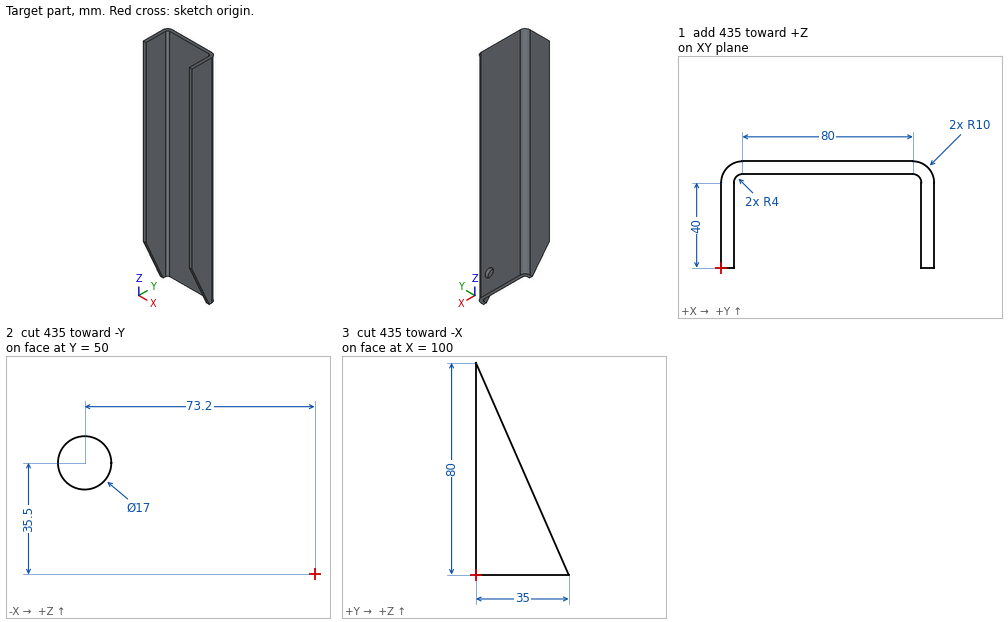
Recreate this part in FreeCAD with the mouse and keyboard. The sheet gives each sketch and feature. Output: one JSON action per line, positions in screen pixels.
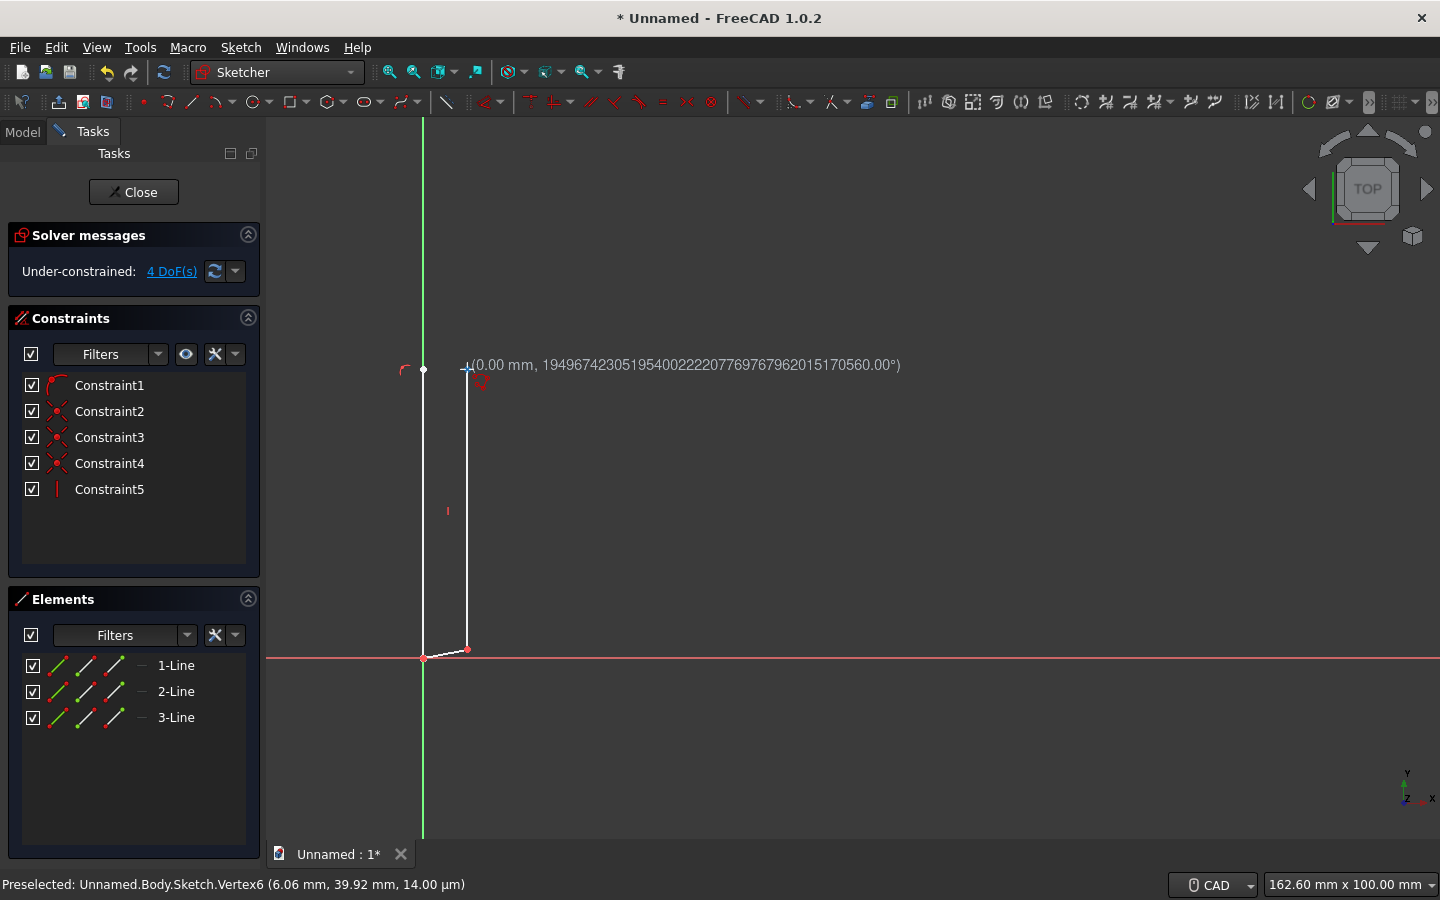
{"action": "left_click", "coordinate": [192, 102]}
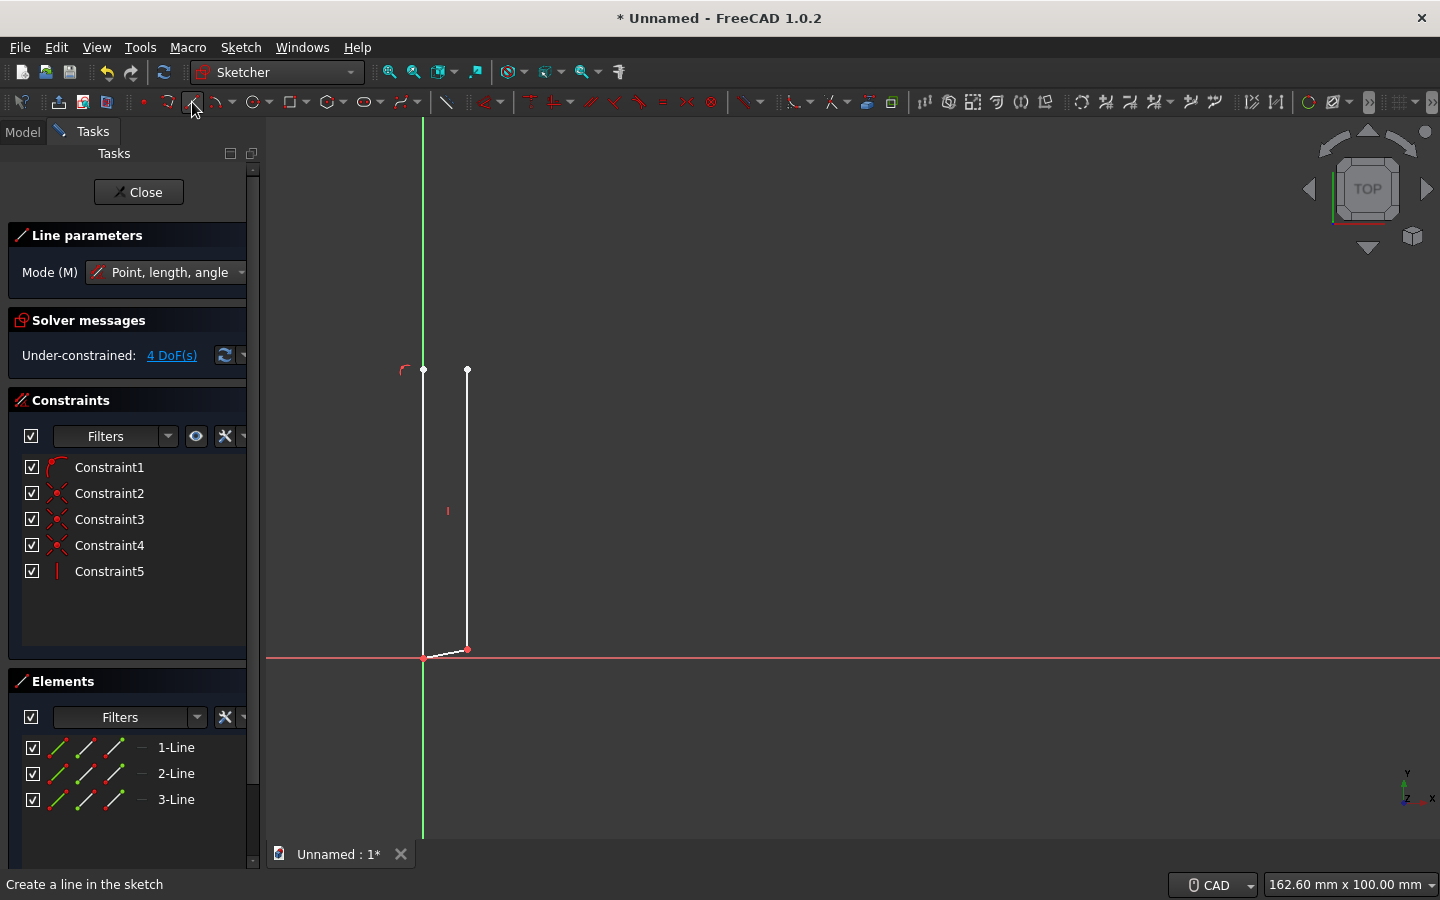
{"action": "left_click", "coordinate": [495, 341]}
{"action": "left_click", "coordinate": [1073, 341]}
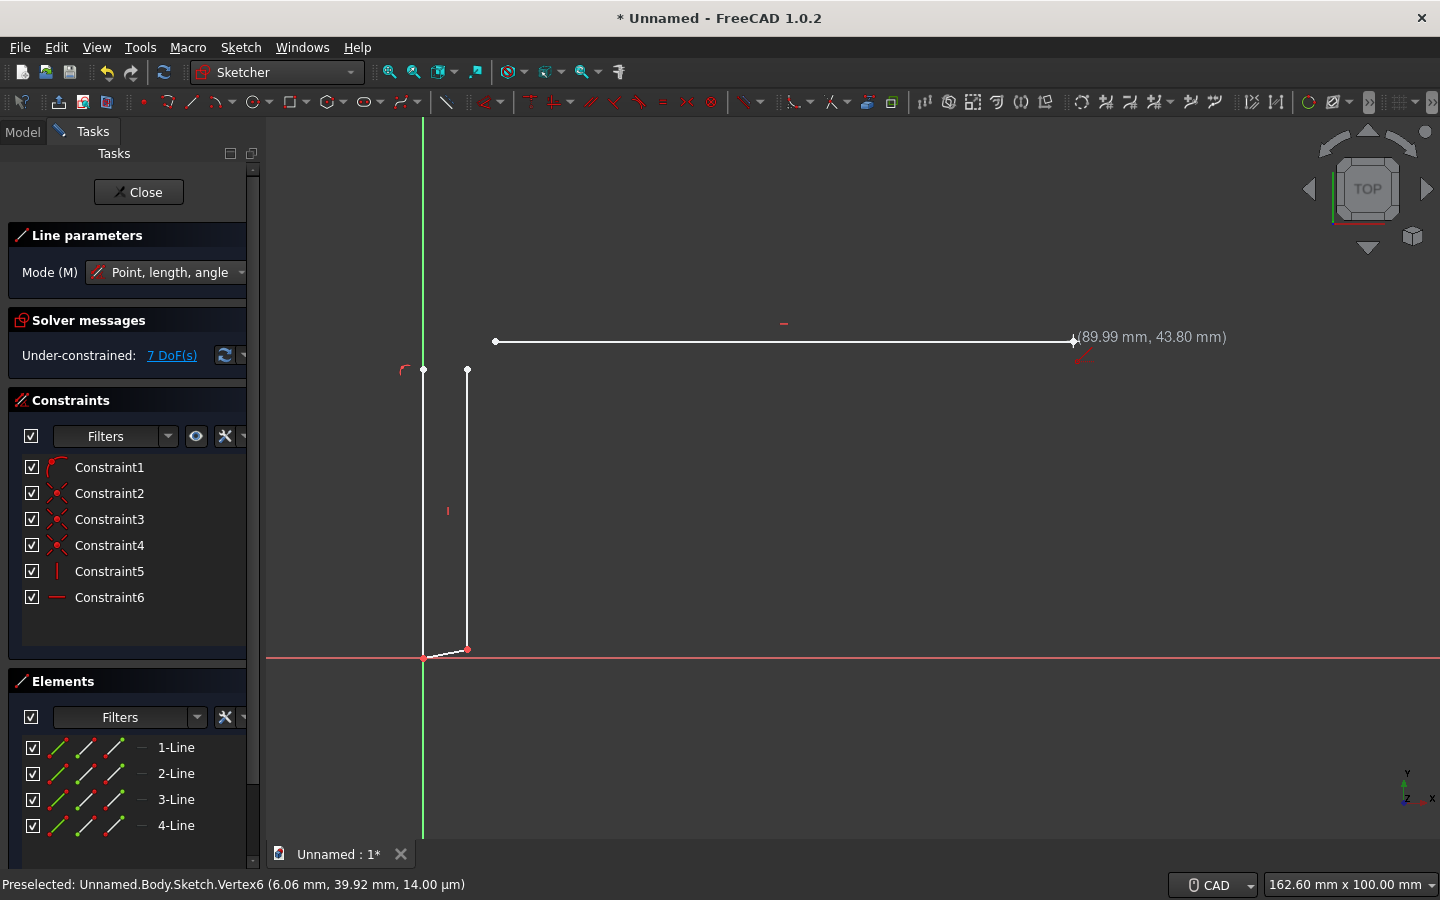
{"action": "left_click", "coordinate": [168, 102]}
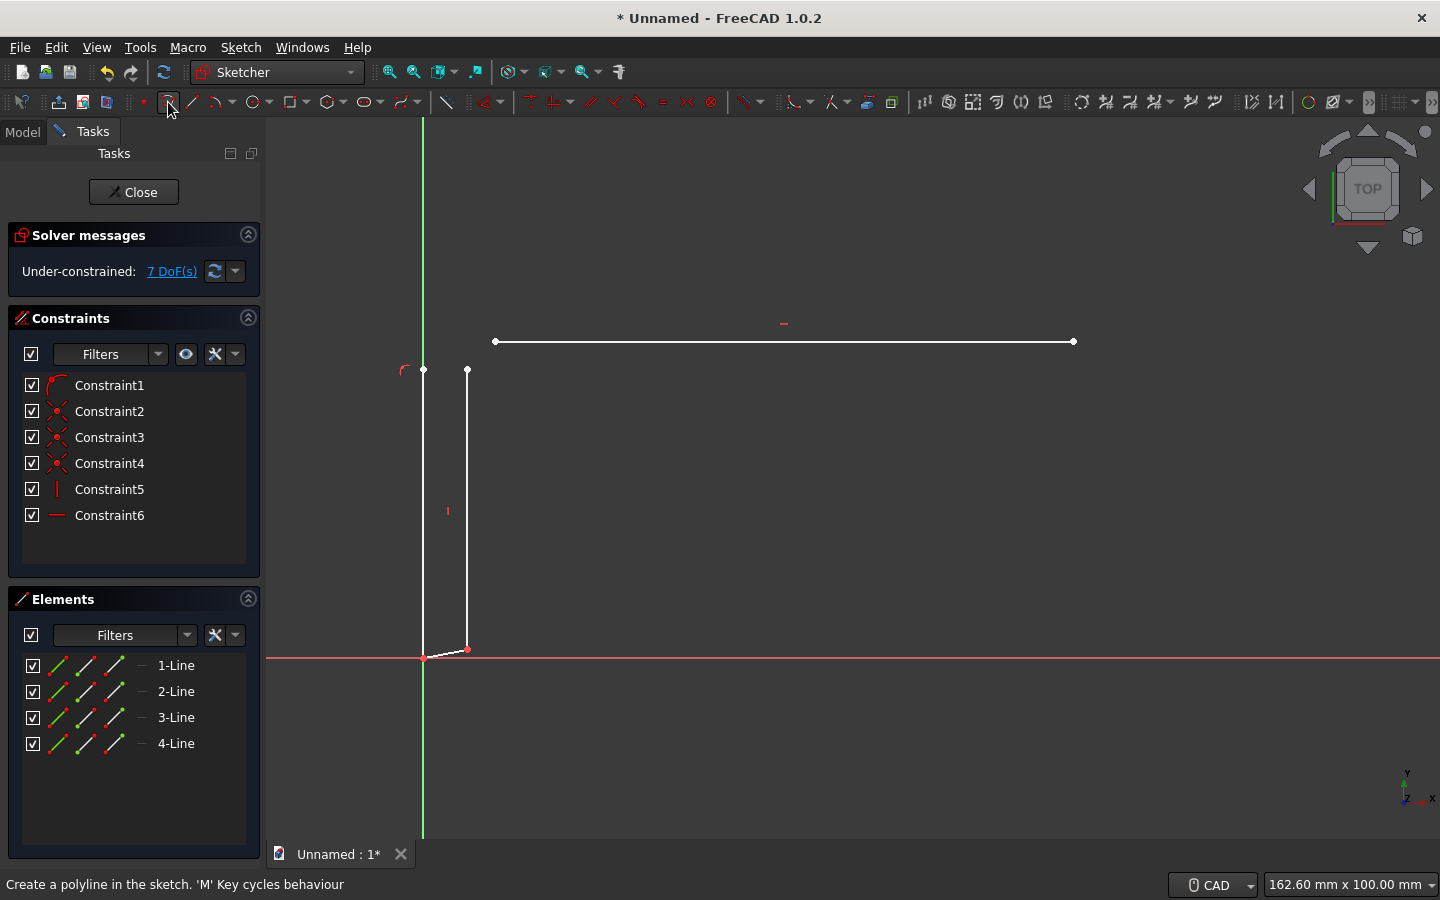
{"action": "left_click", "coordinate": [1102, 369]}
{"action": "left_click", "coordinate": [1102, 658]}
{"action": "left_click", "coordinate": [1145, 649]}
{"action": "left_click", "coordinate": [1145, 369]}
{"action": "right_click", "coordinate": [1145, 369]}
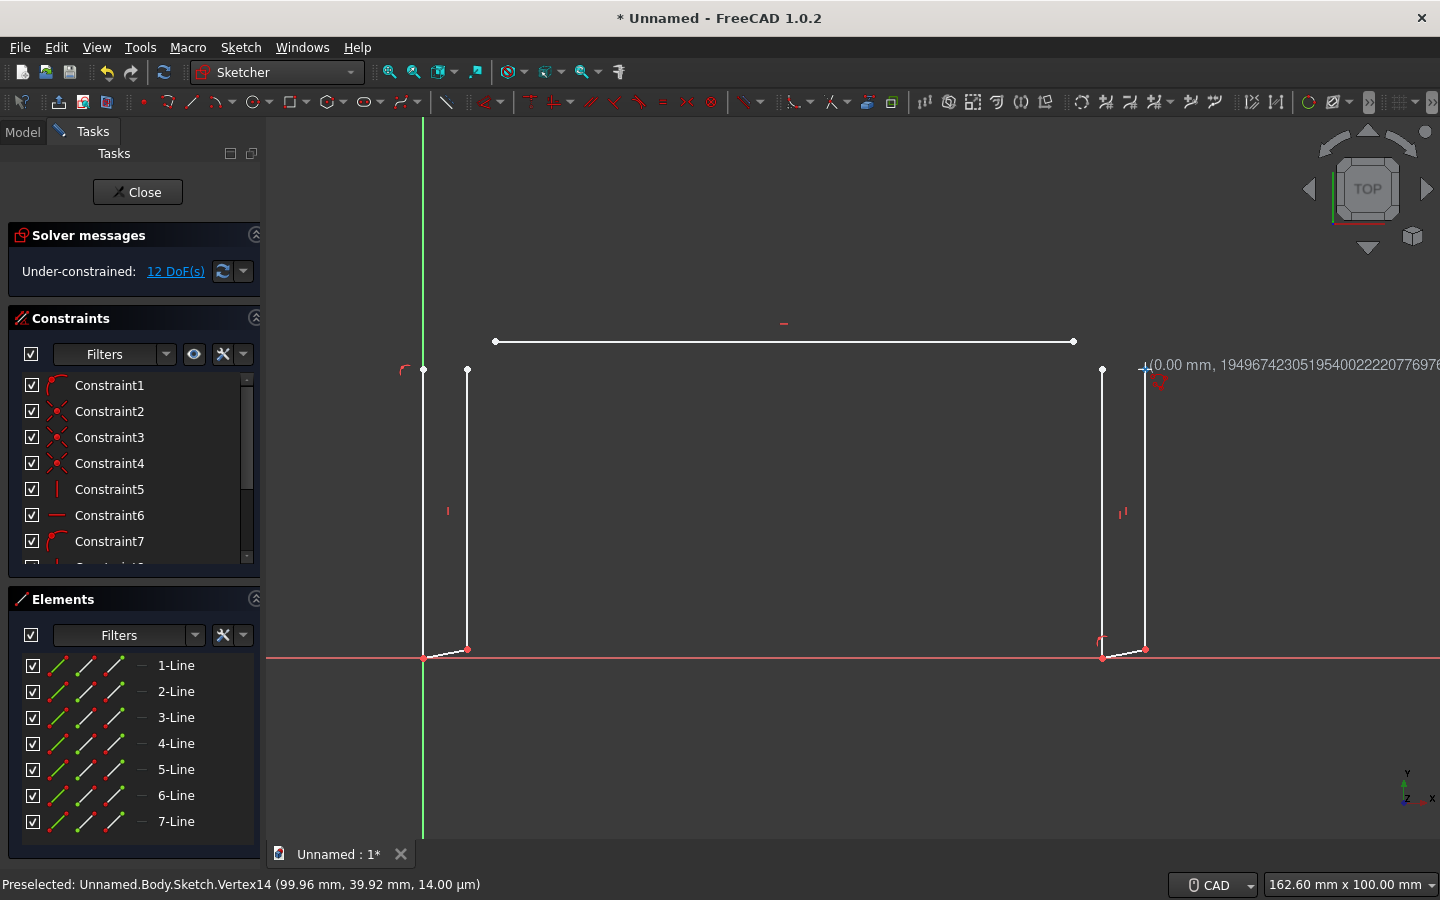
{"action": "left_click", "coordinate": [192, 102]}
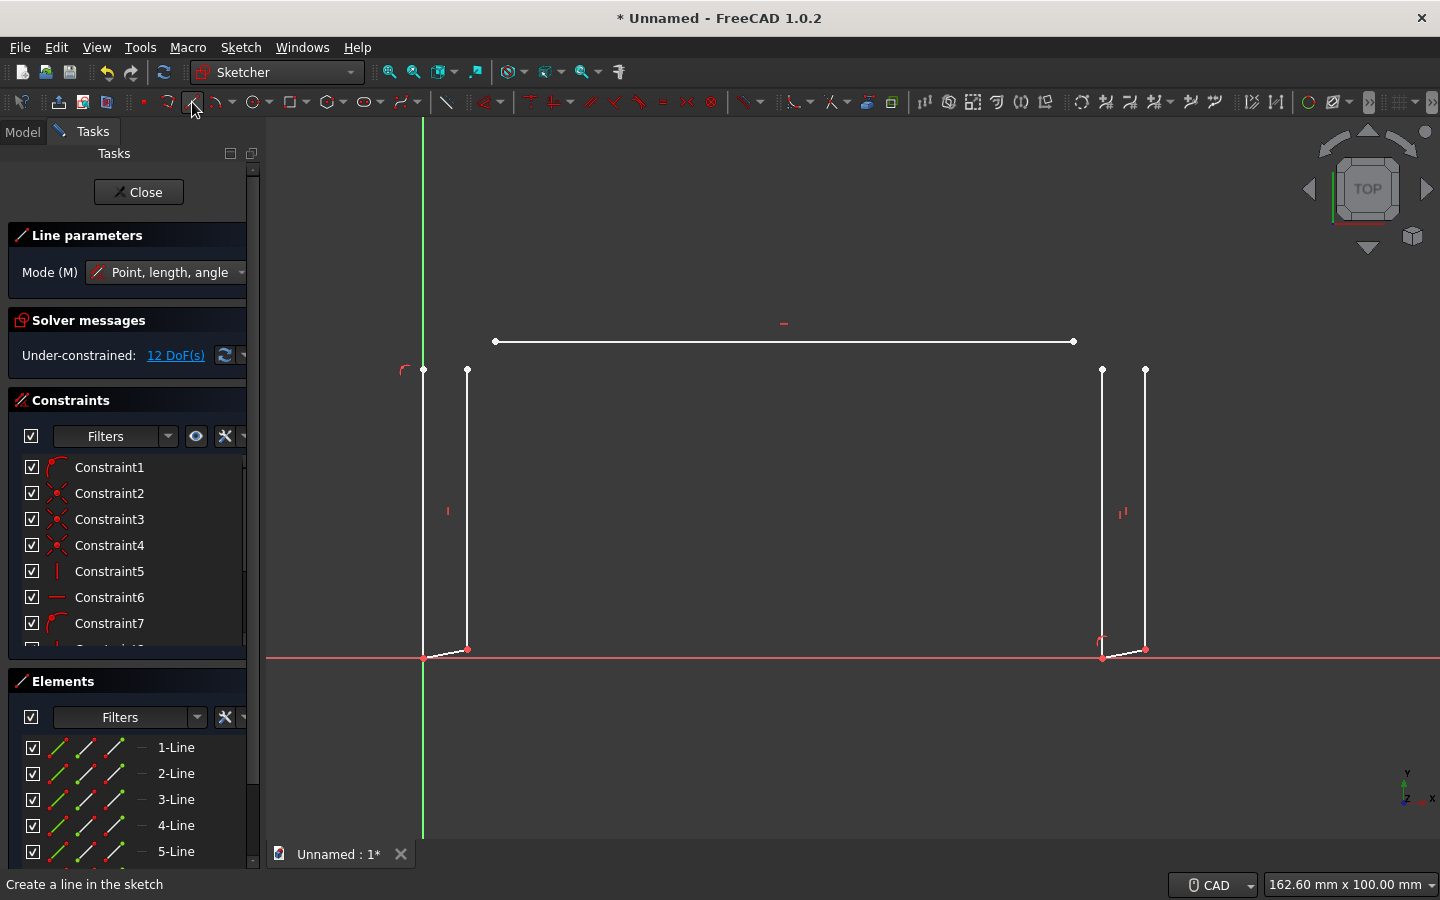
{"action": "left_click", "coordinate": [1073, 297]}
{"action": "left_click", "coordinate": [495, 297]}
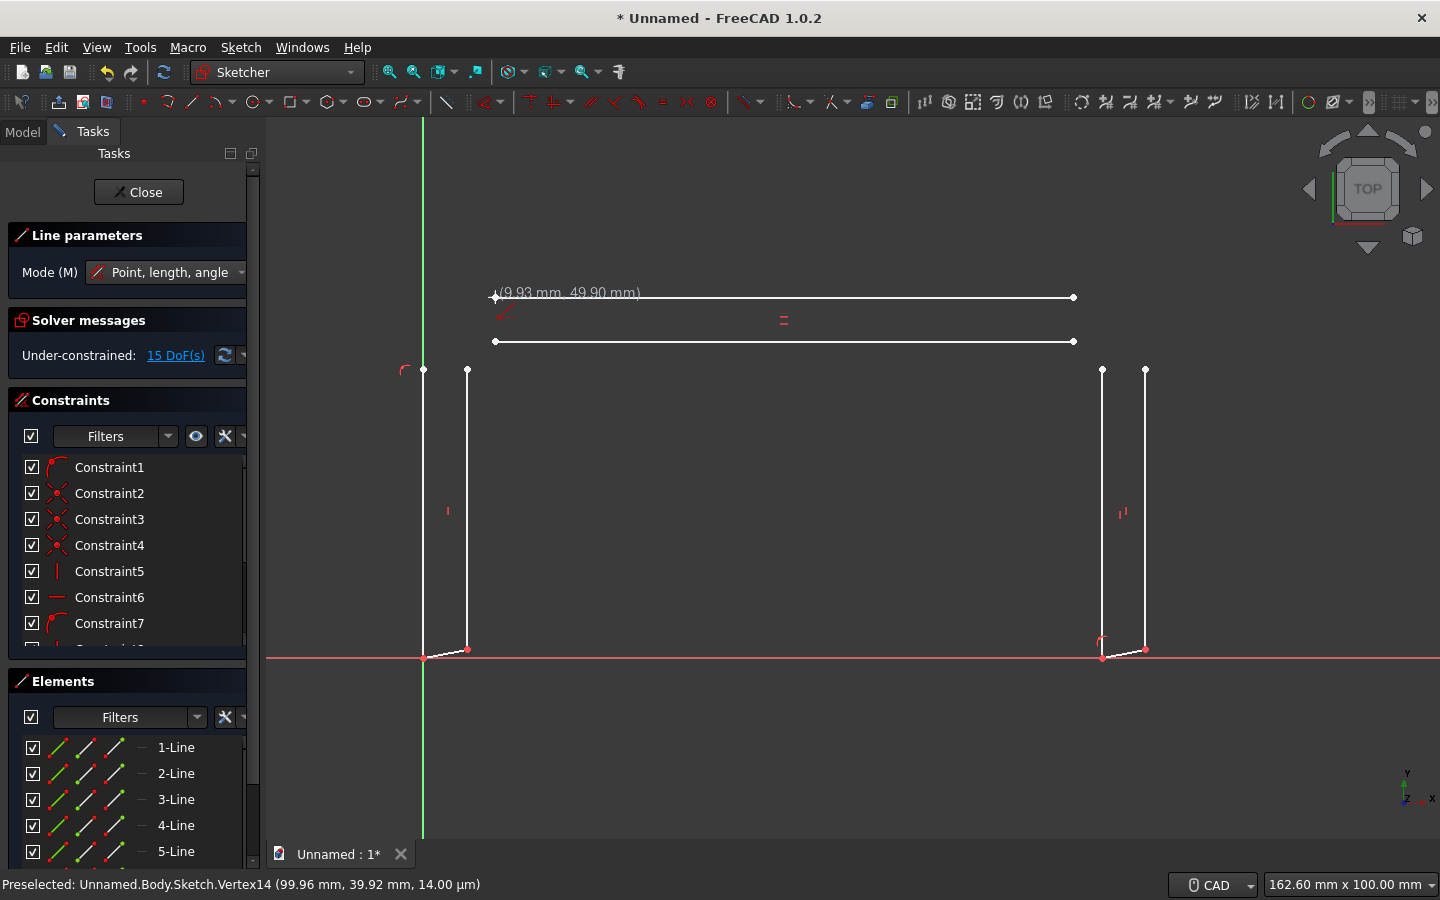
{"action": "left_click", "coordinate": [234, 102]}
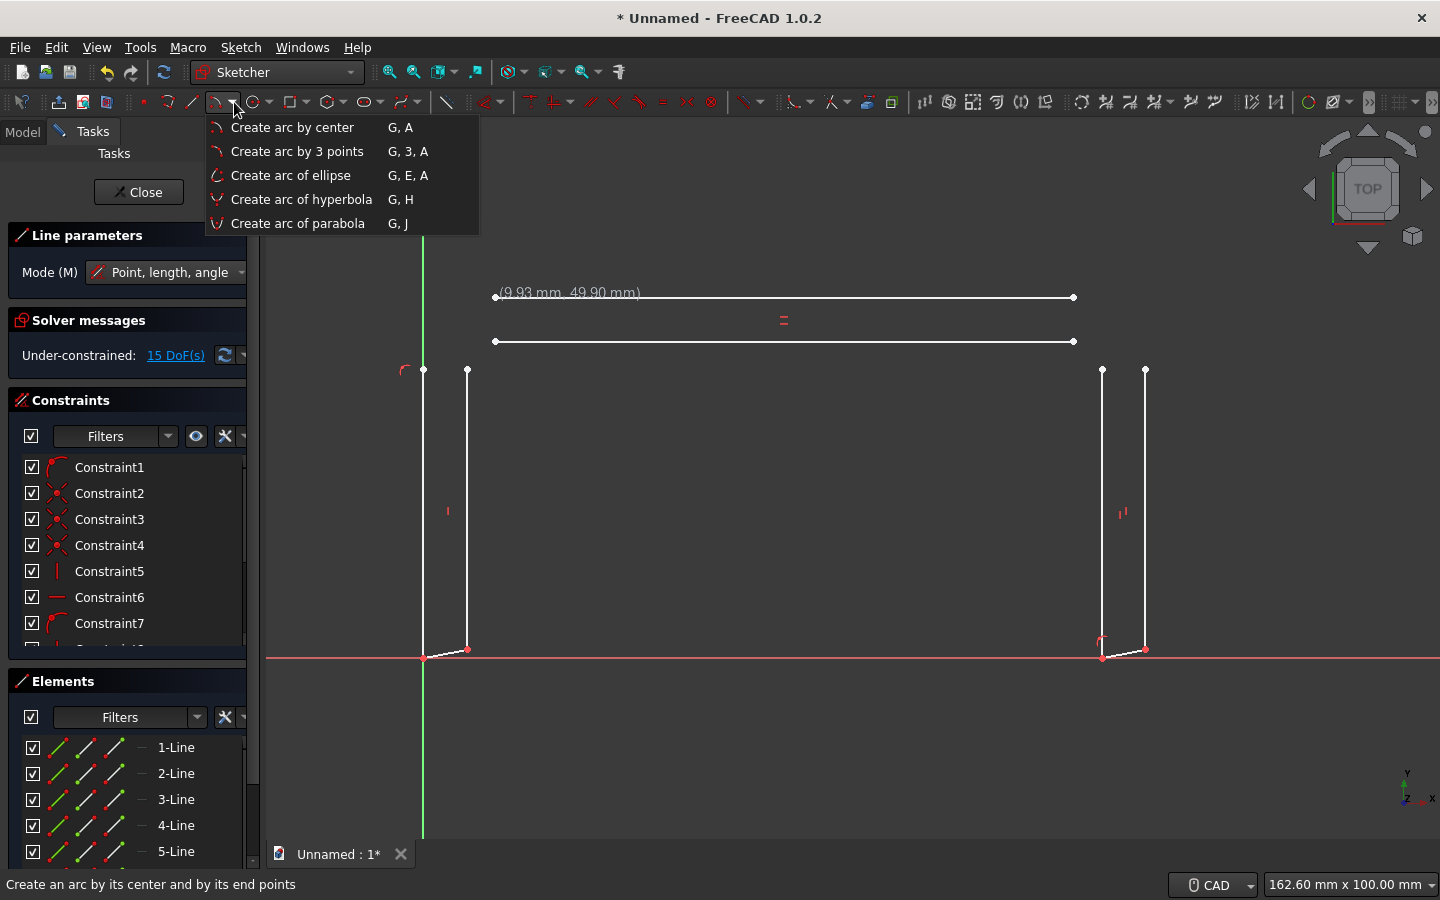
{"action": "left_click", "coordinate": [342, 151]}